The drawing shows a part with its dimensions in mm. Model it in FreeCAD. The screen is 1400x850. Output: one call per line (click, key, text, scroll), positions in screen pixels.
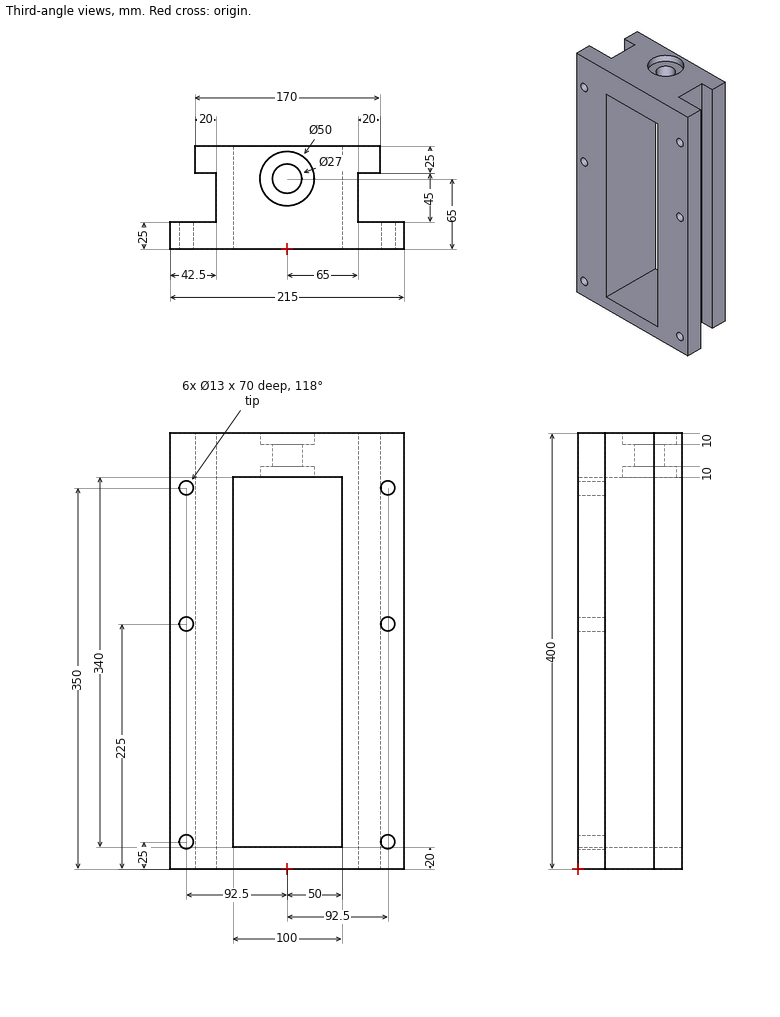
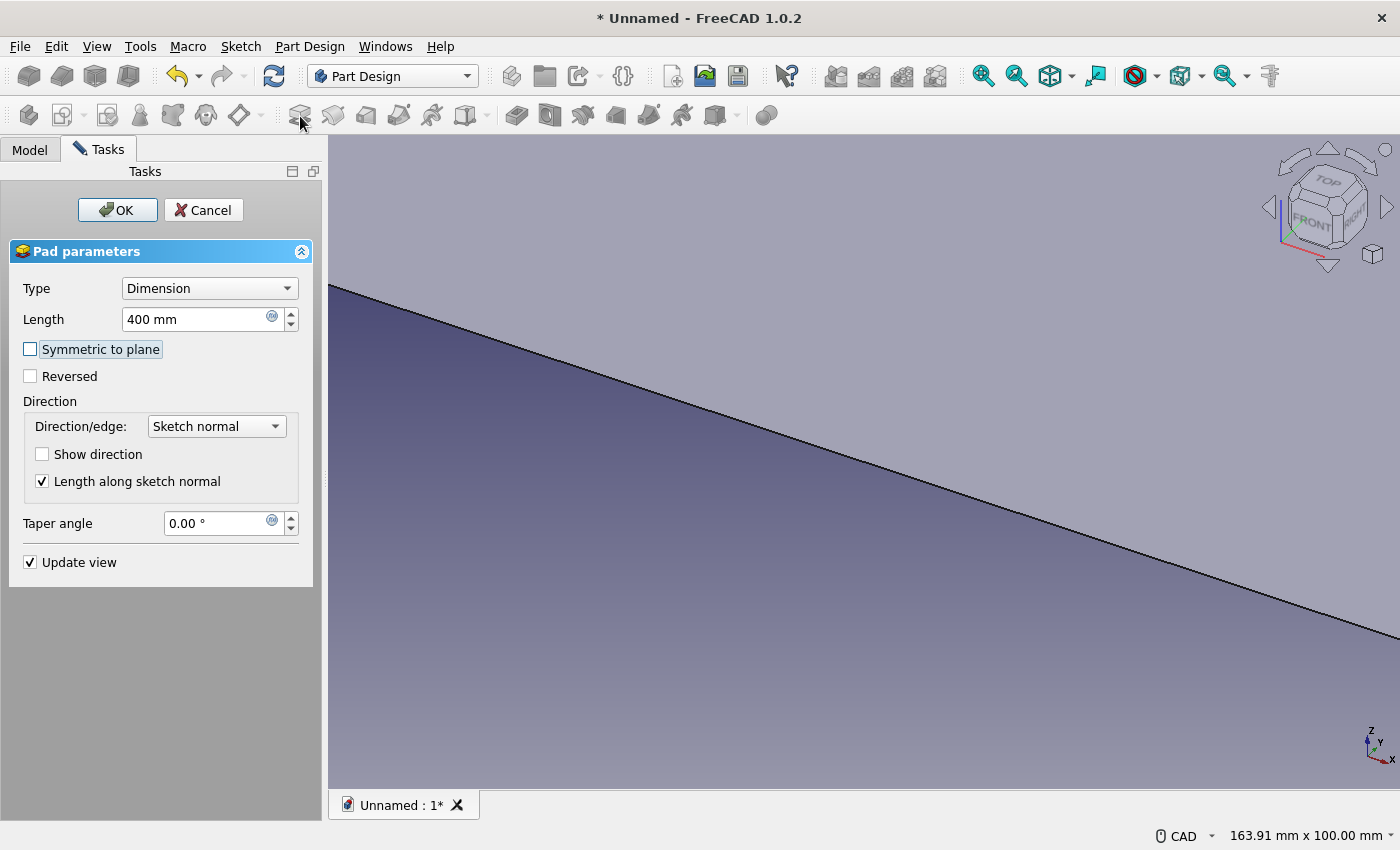
click(118, 210)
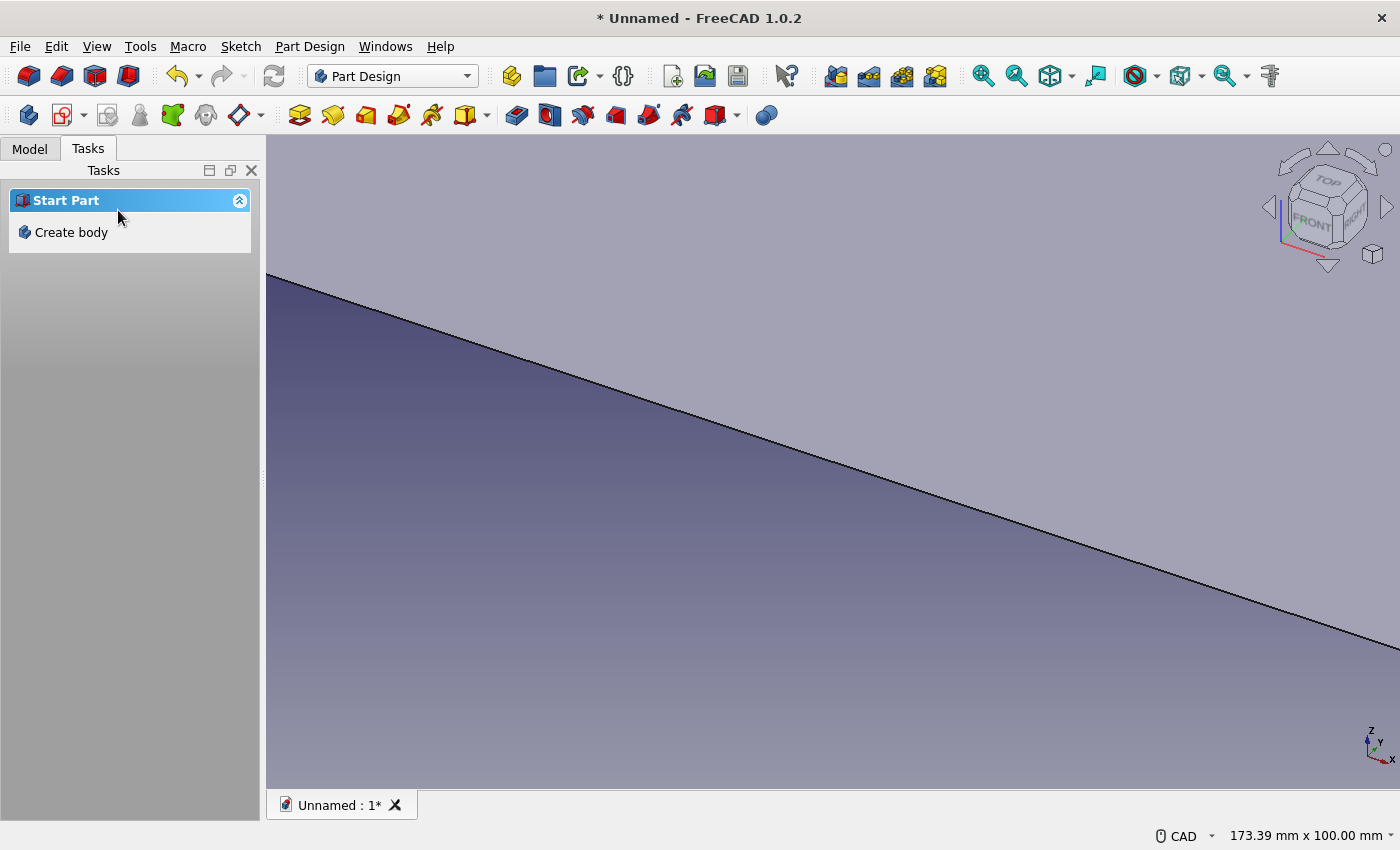
click(984, 76)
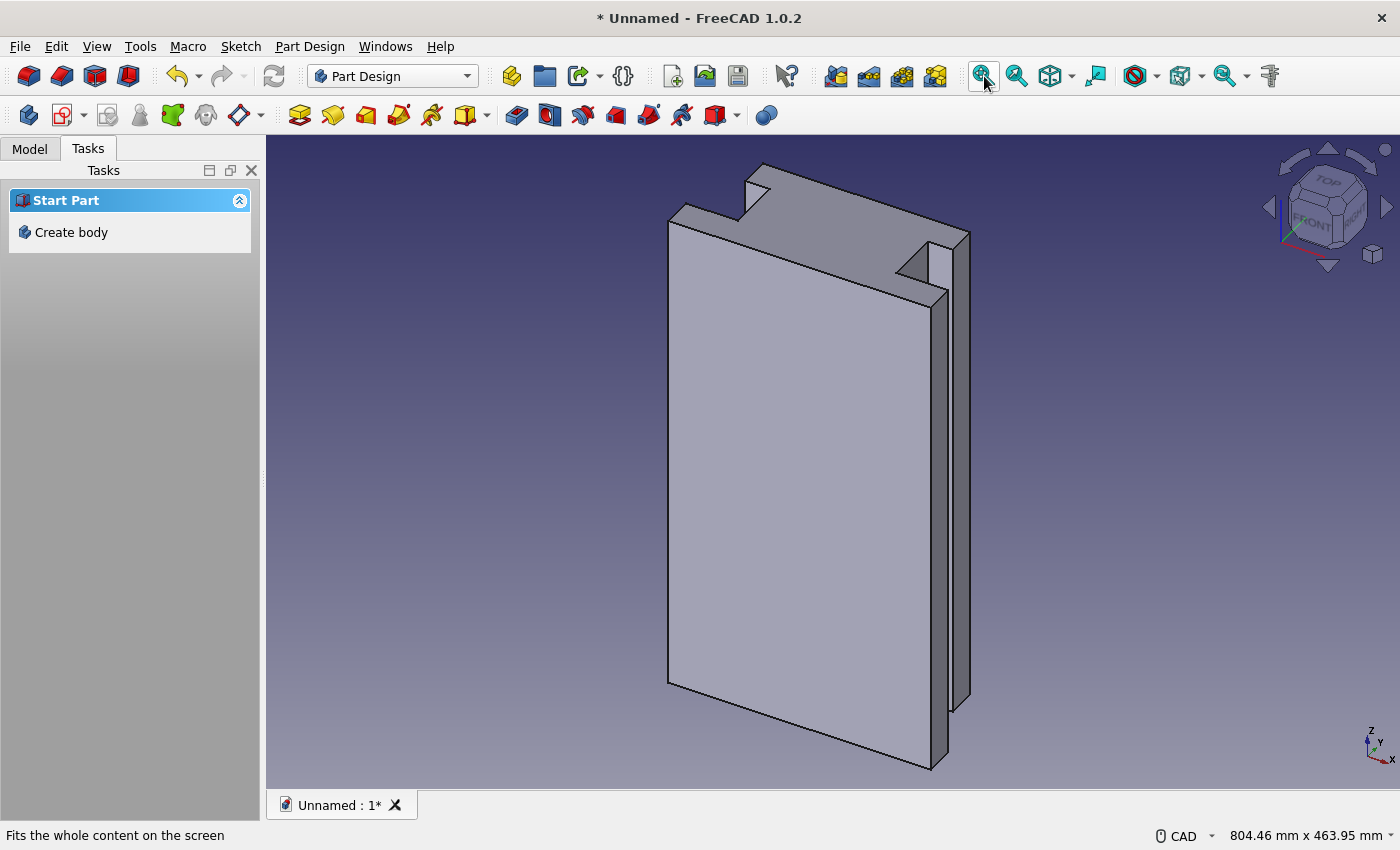
key(4)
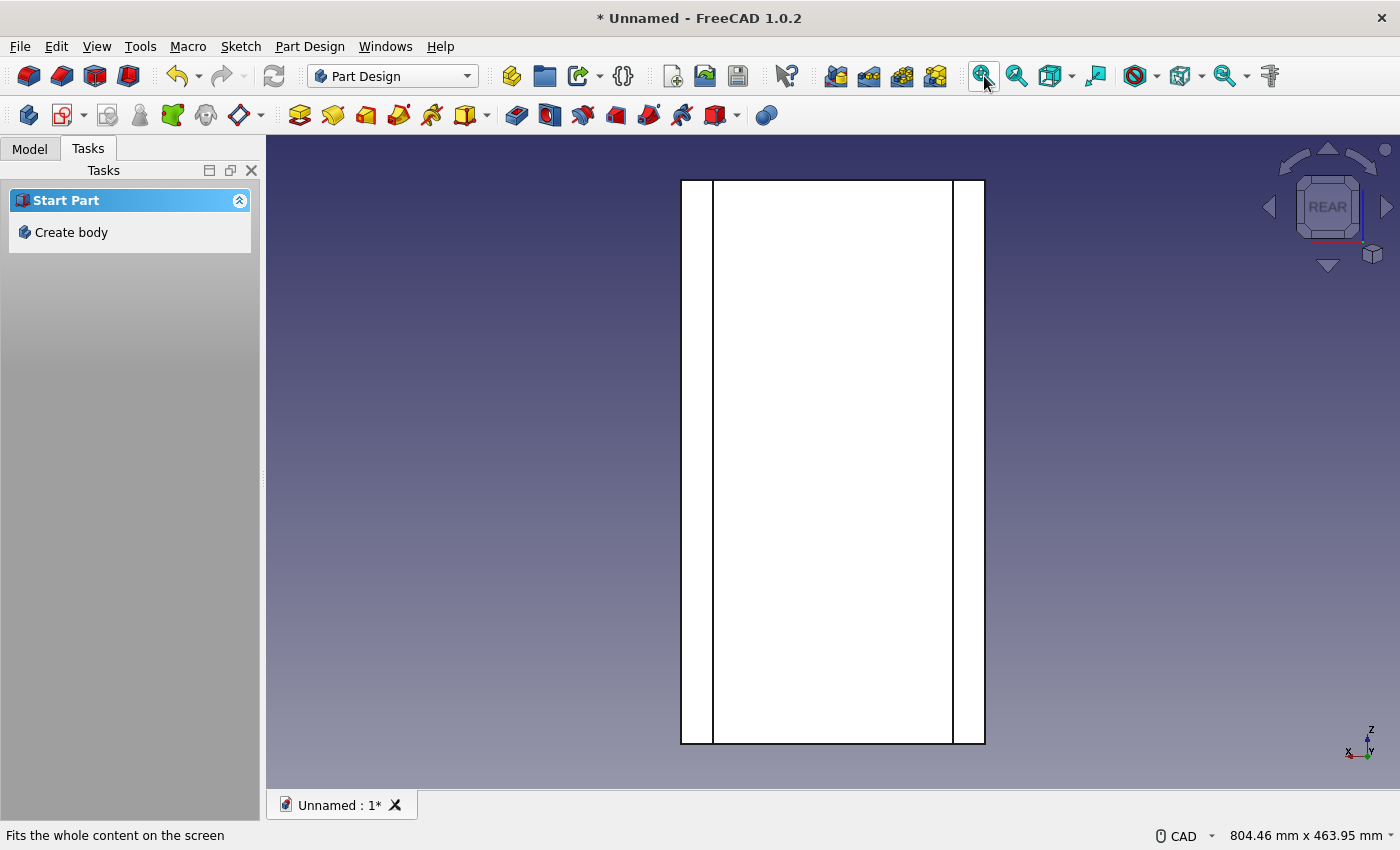
click(833, 300)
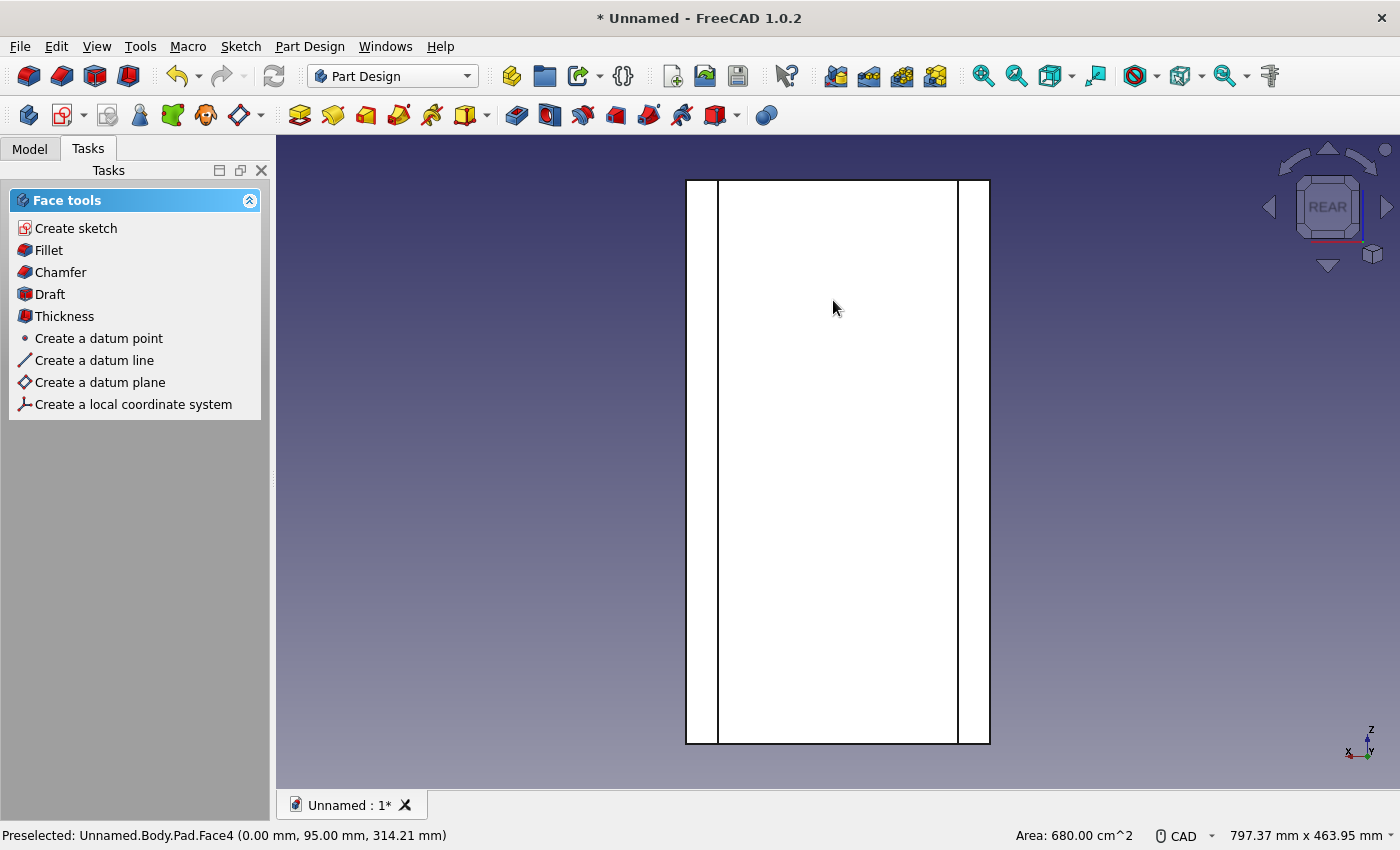
click(62, 116)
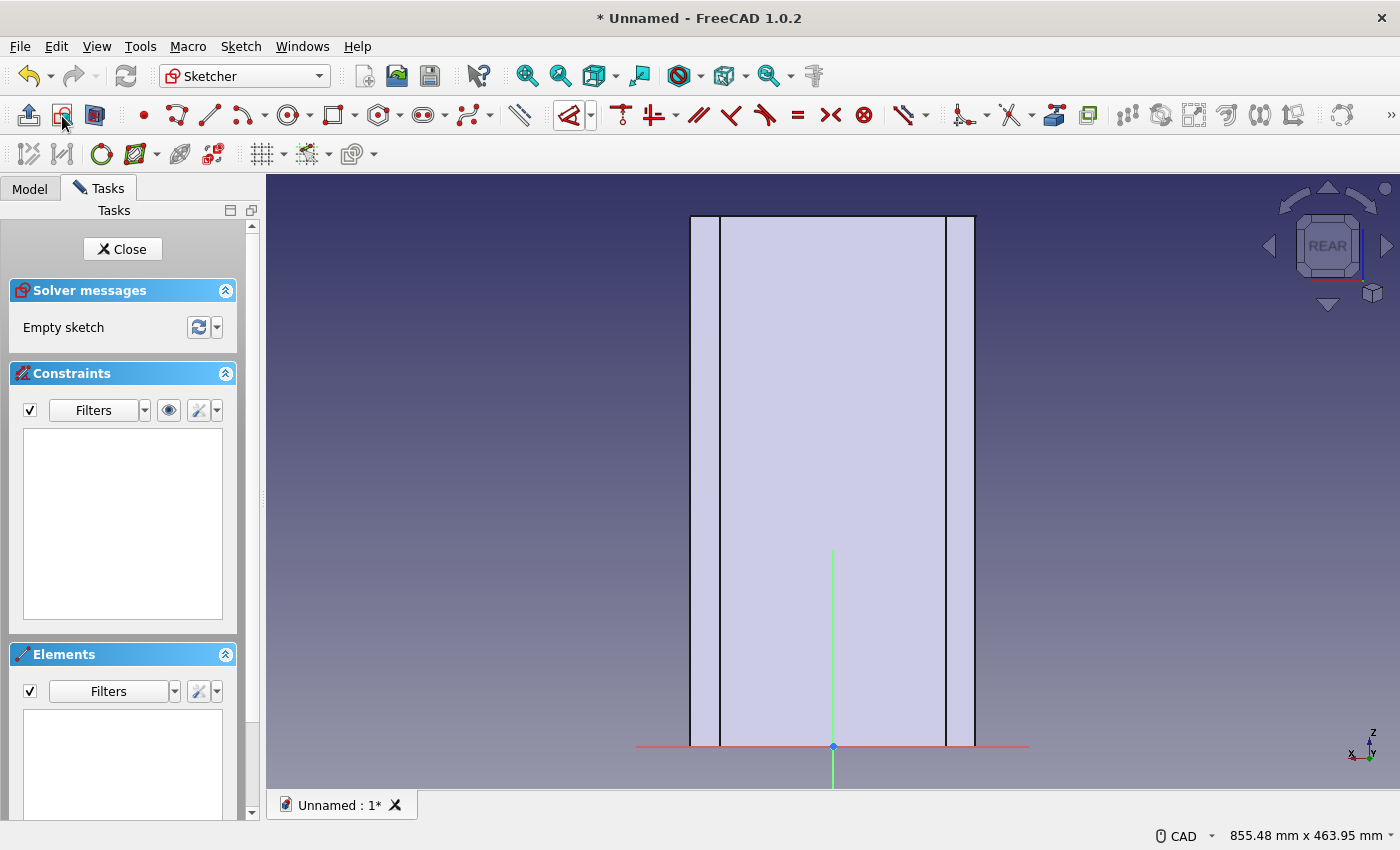
scroll(455, 362, down, 1)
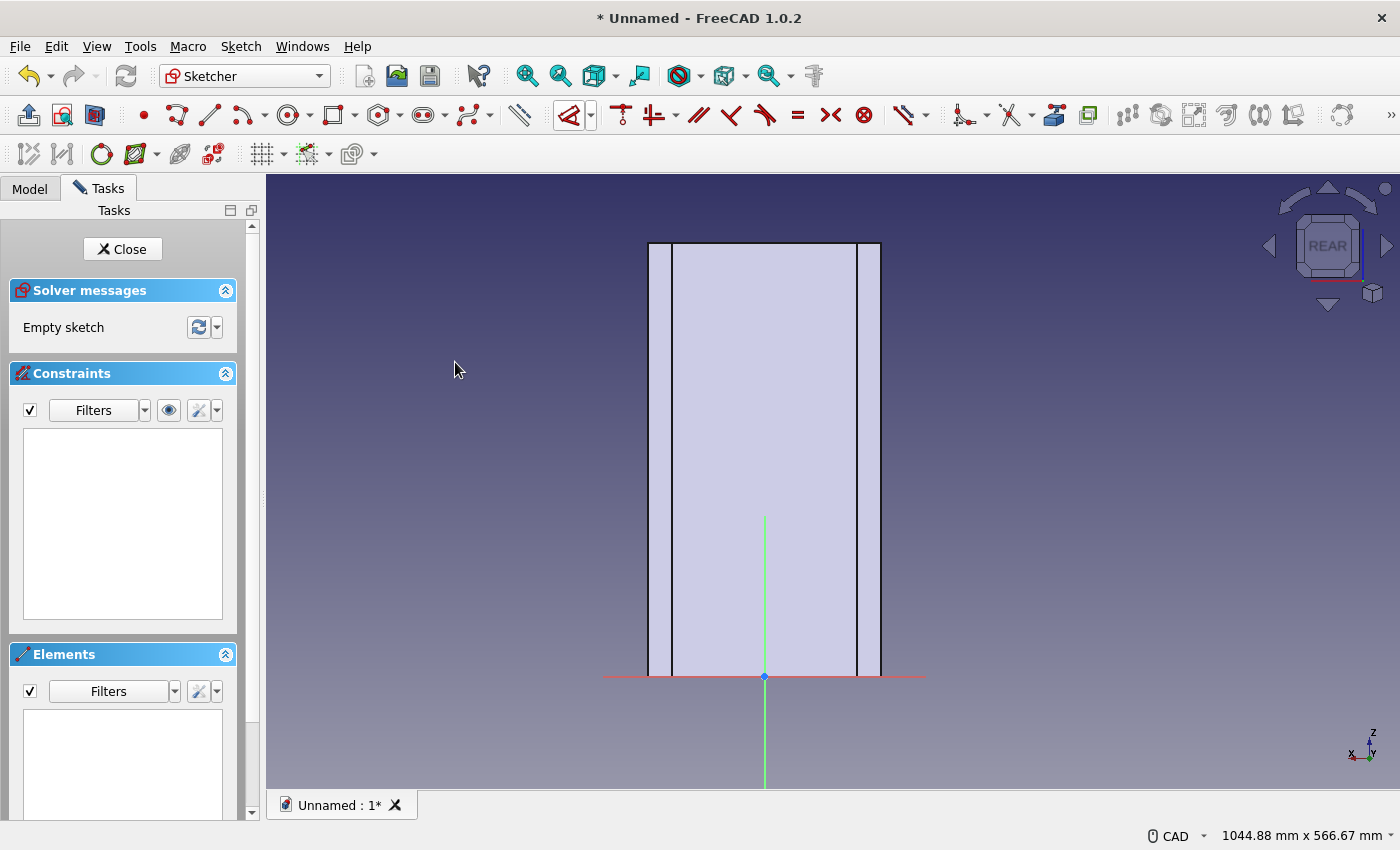
key(g)
key(r)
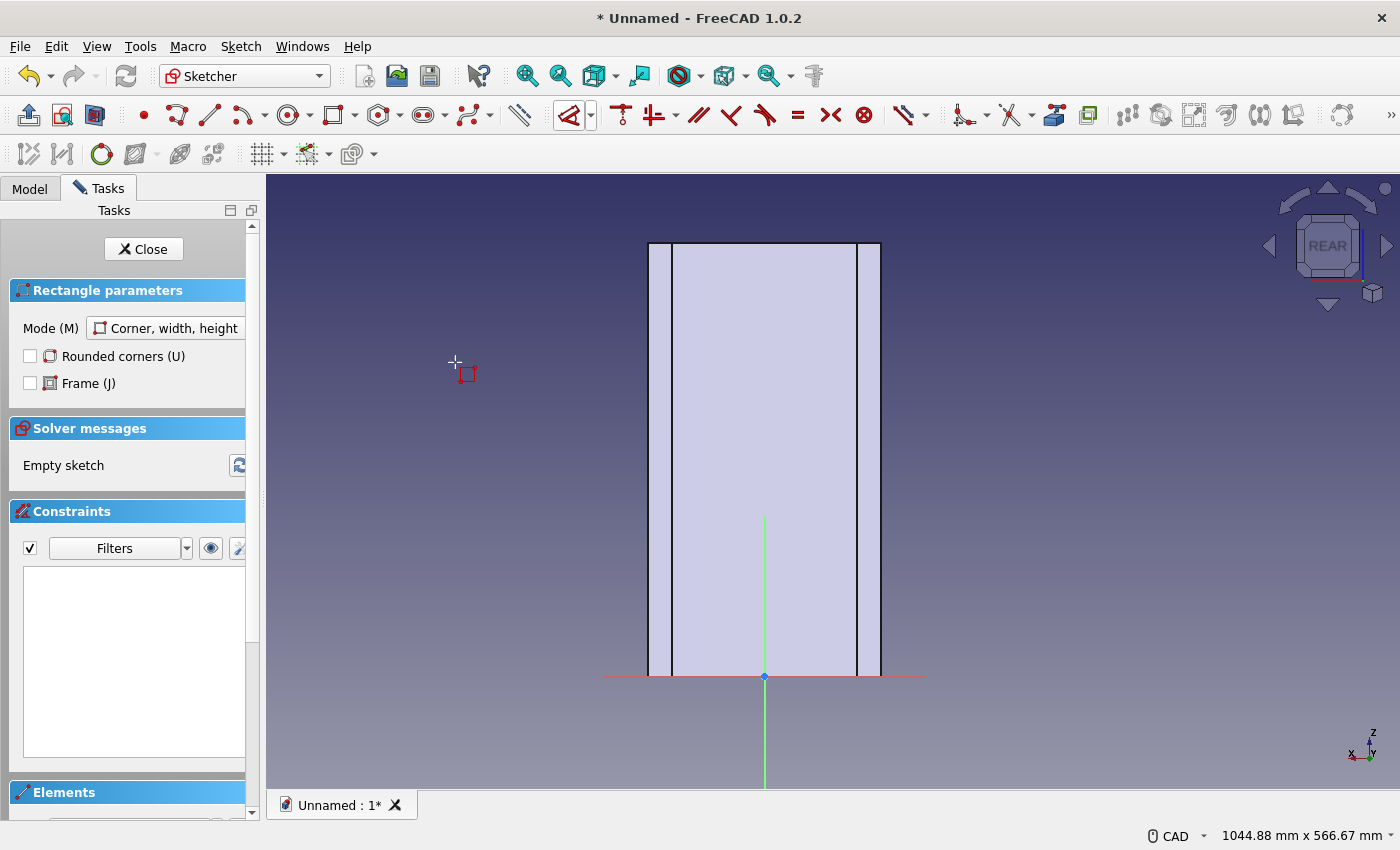
click(710, 286)
move(819, 655)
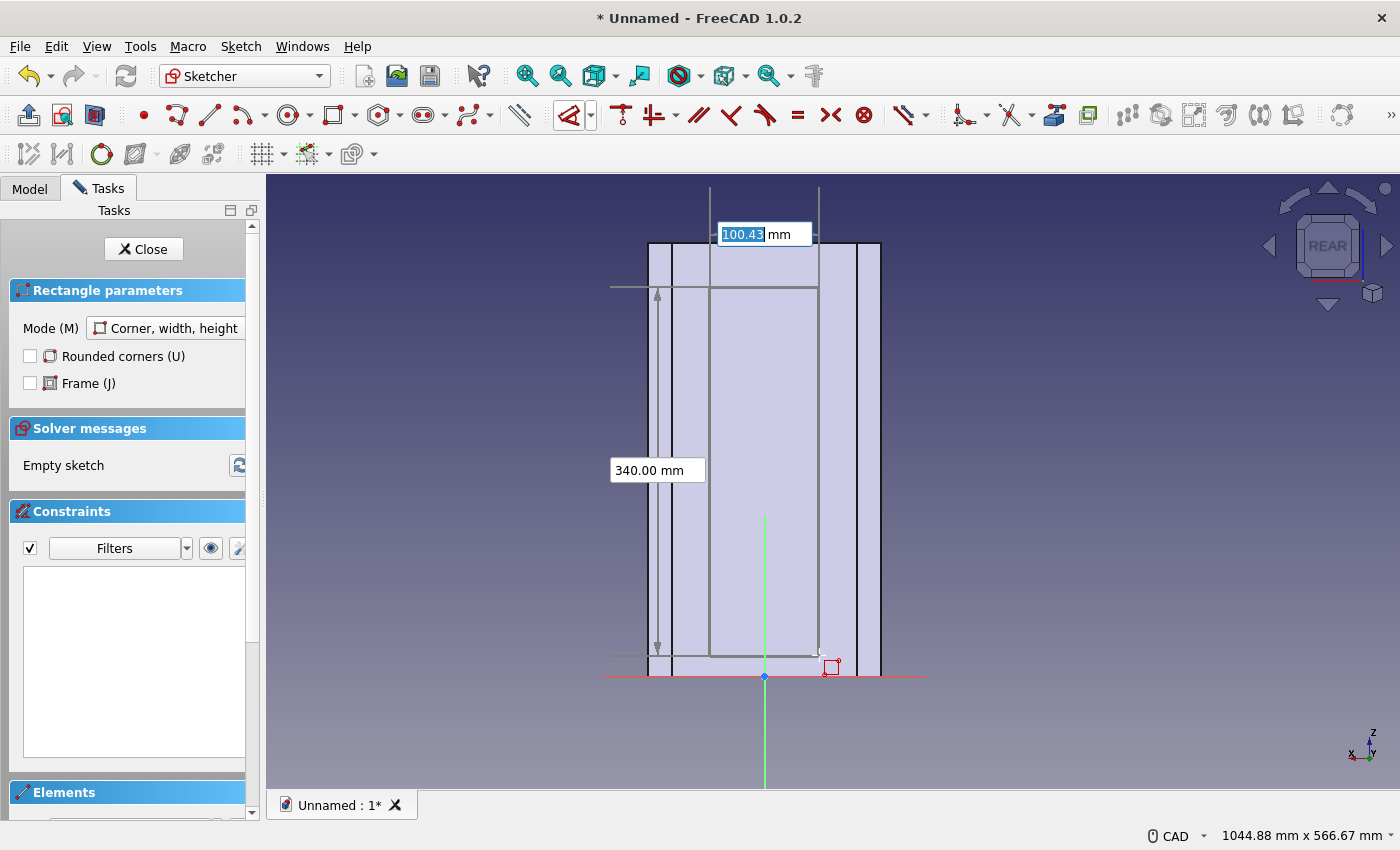
text(100)
key(Tab)
text(340)
key(Return)
key(Escape)